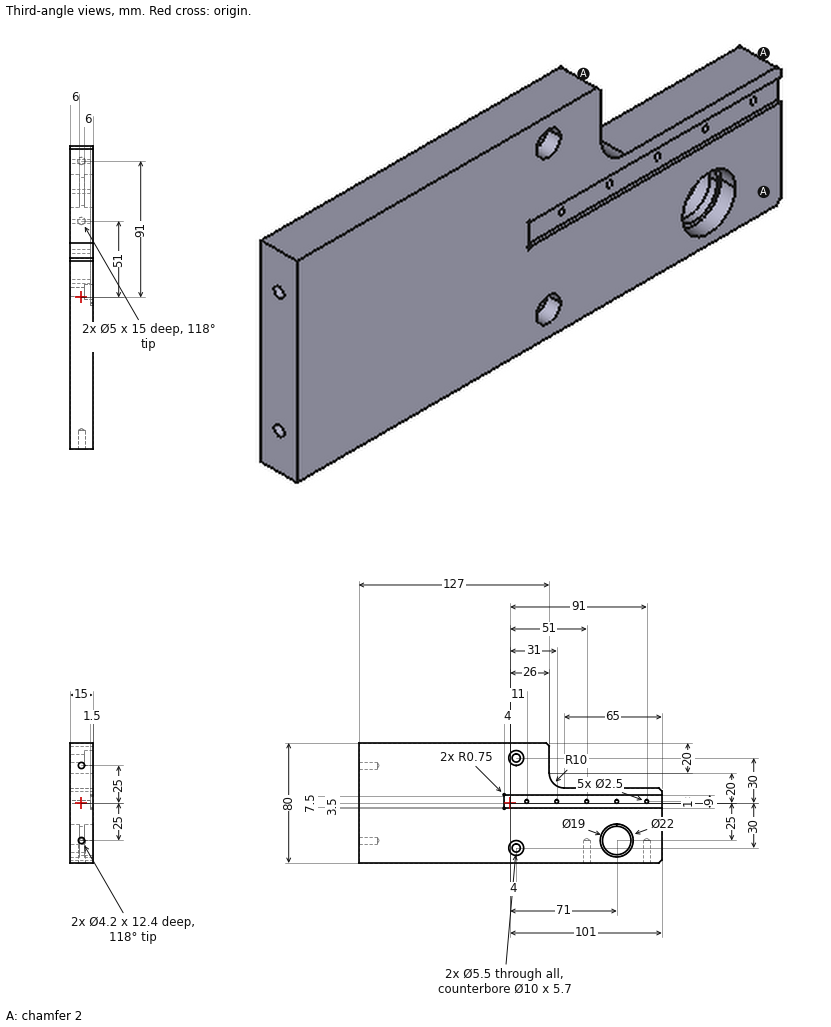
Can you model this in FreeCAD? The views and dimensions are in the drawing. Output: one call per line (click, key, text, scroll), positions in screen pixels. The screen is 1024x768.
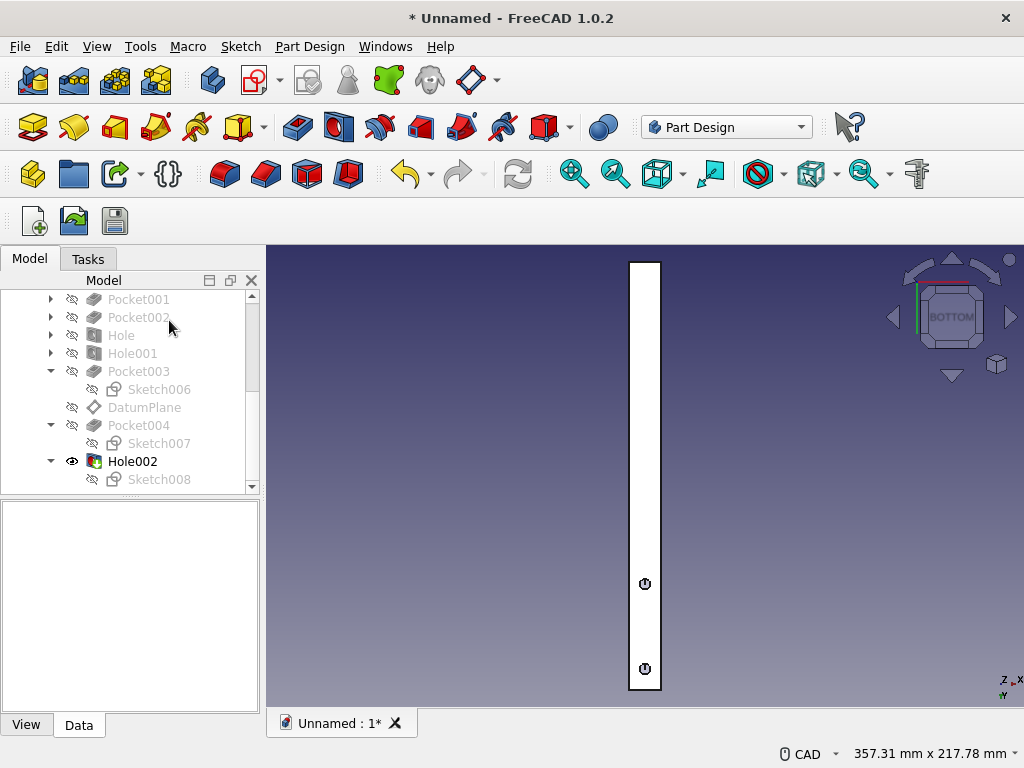
key(0)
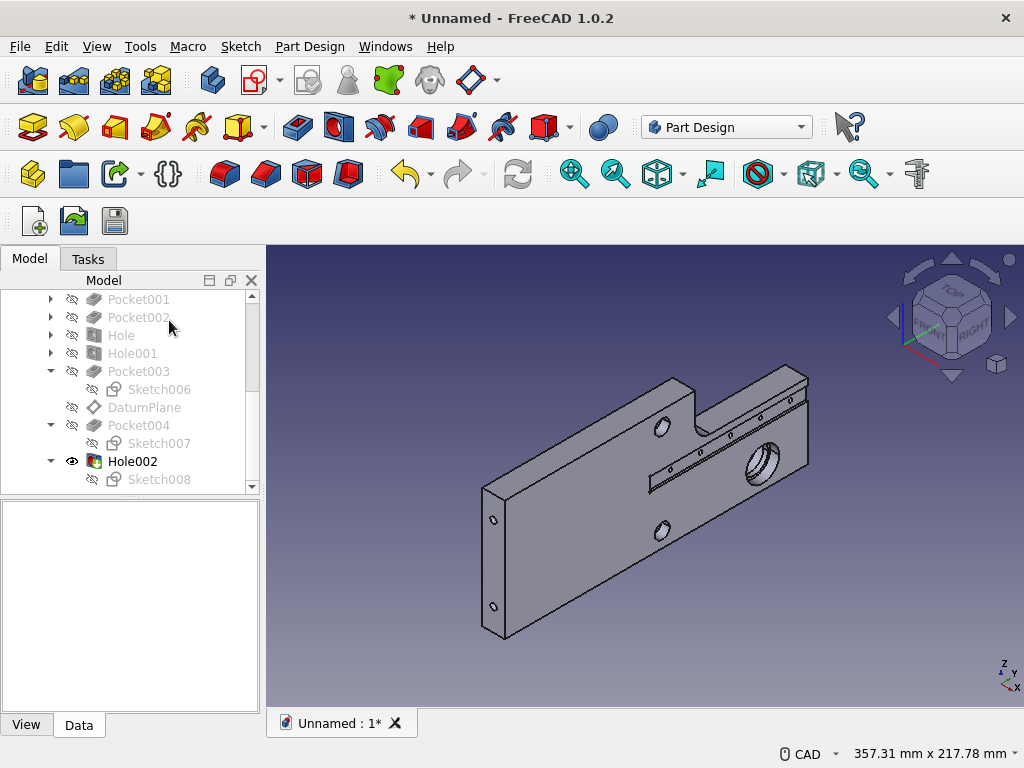
key(2)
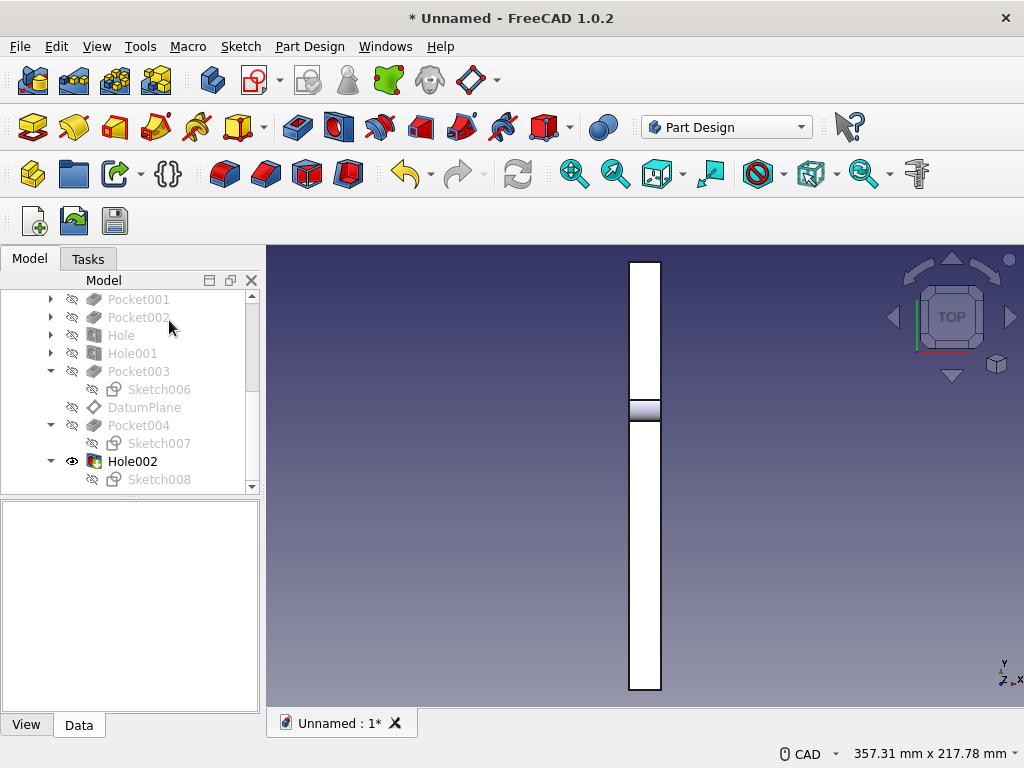
click(645, 420)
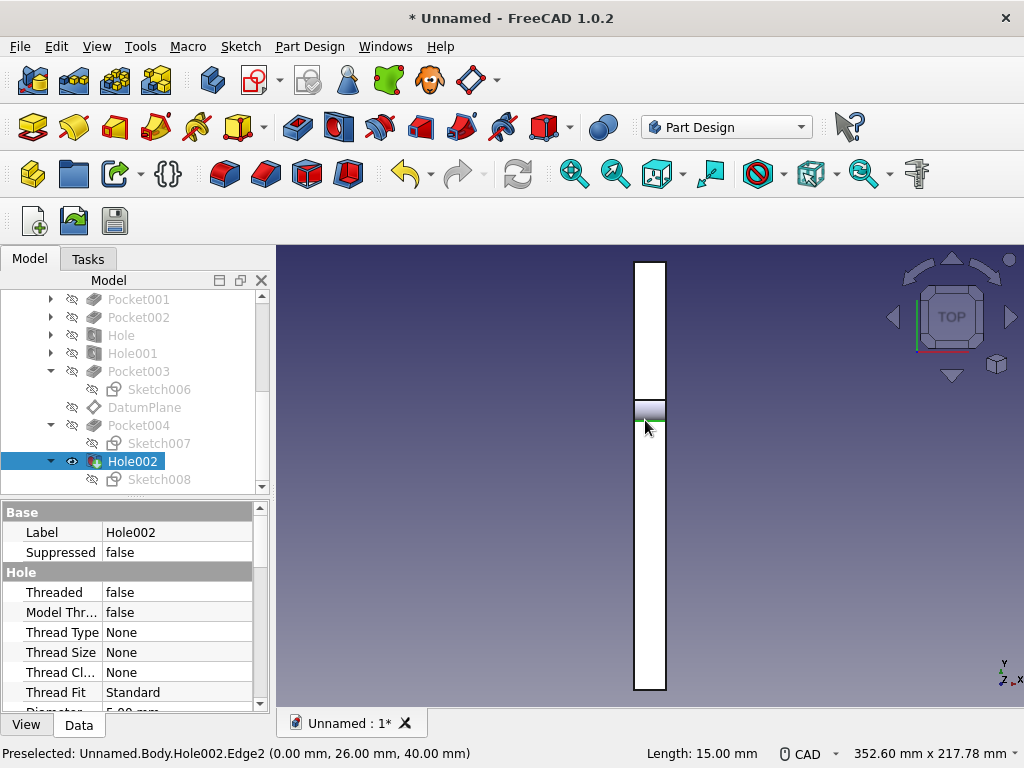
key(1)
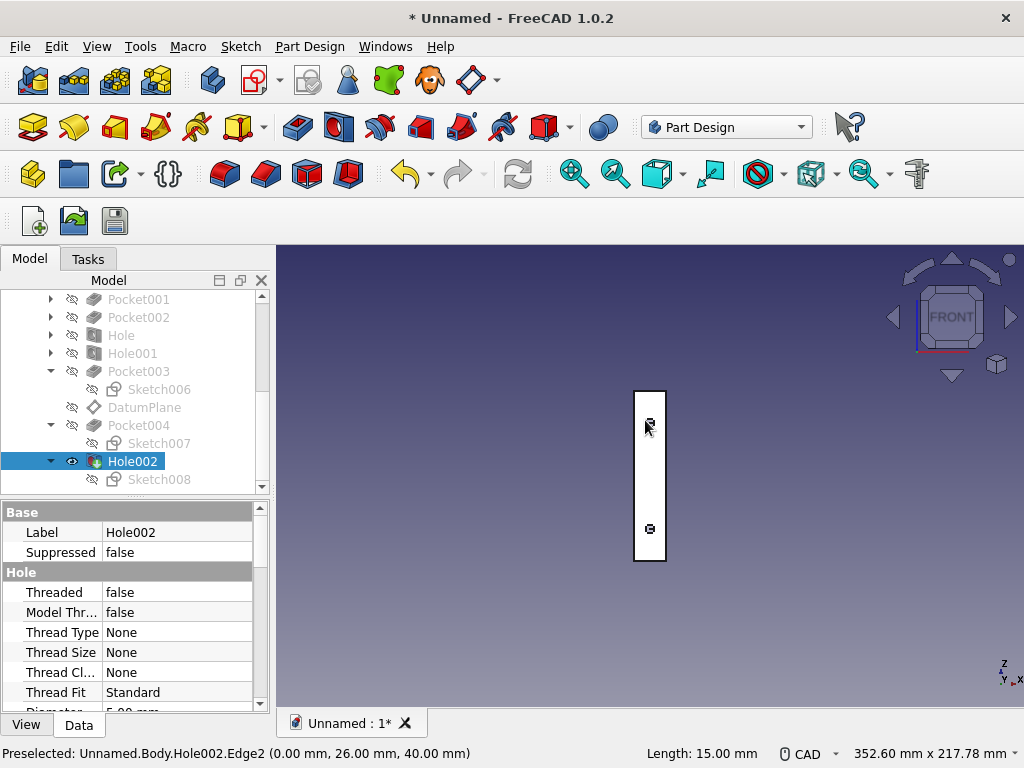
click(575, 174)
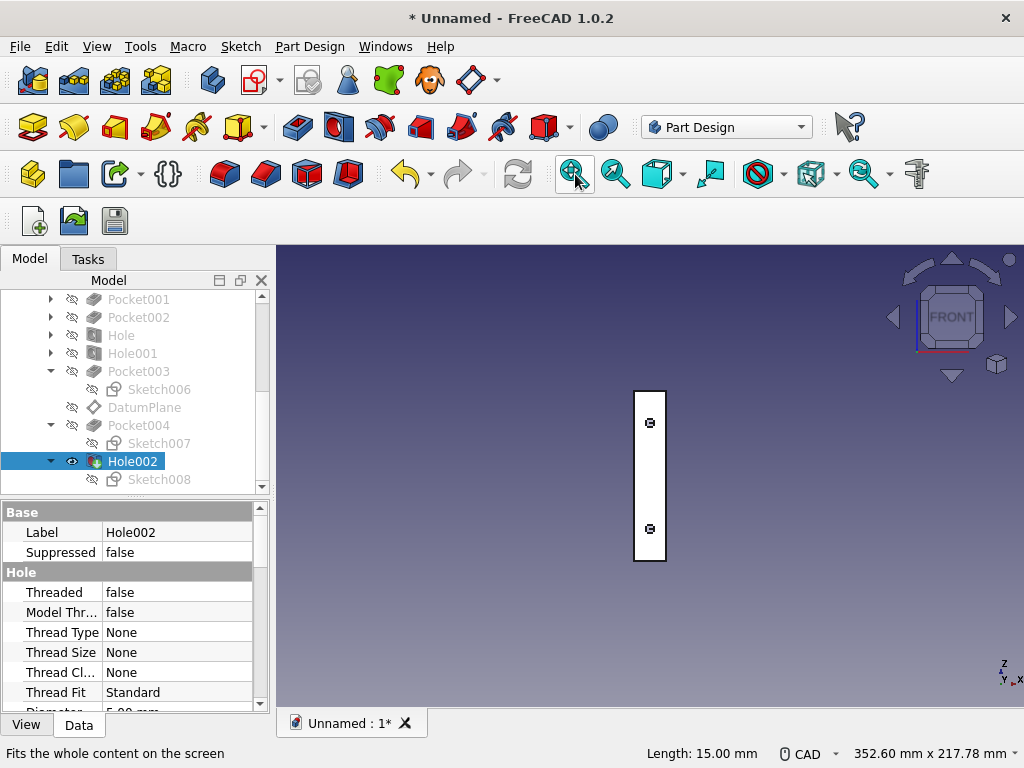
key(3)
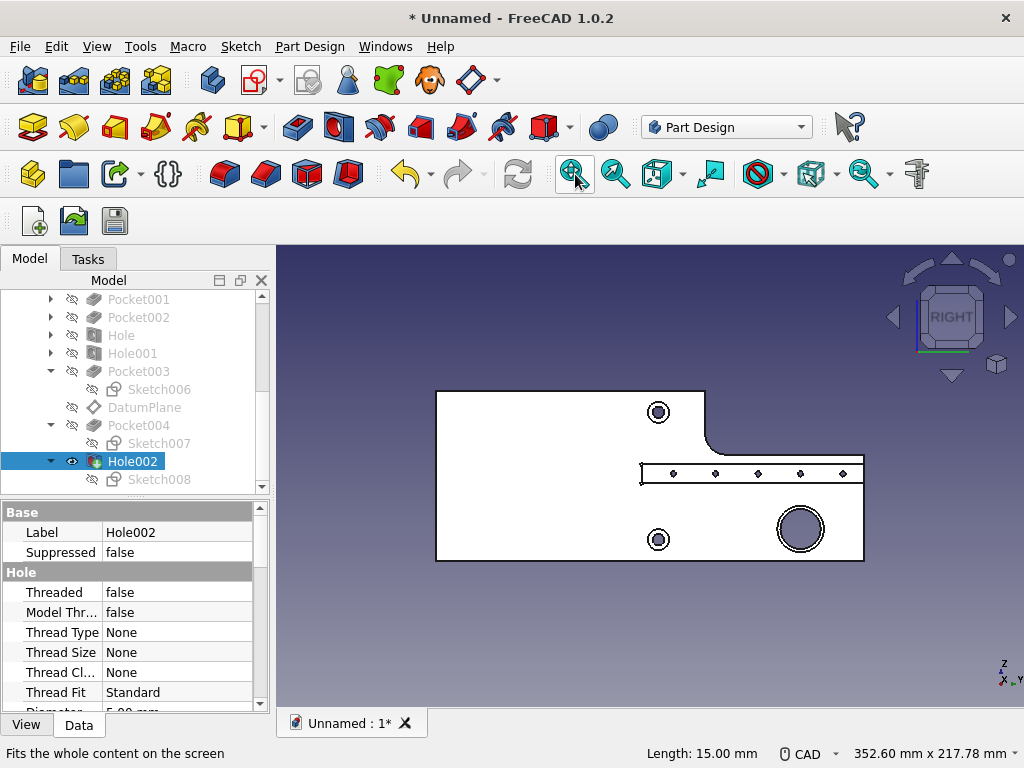
key(5)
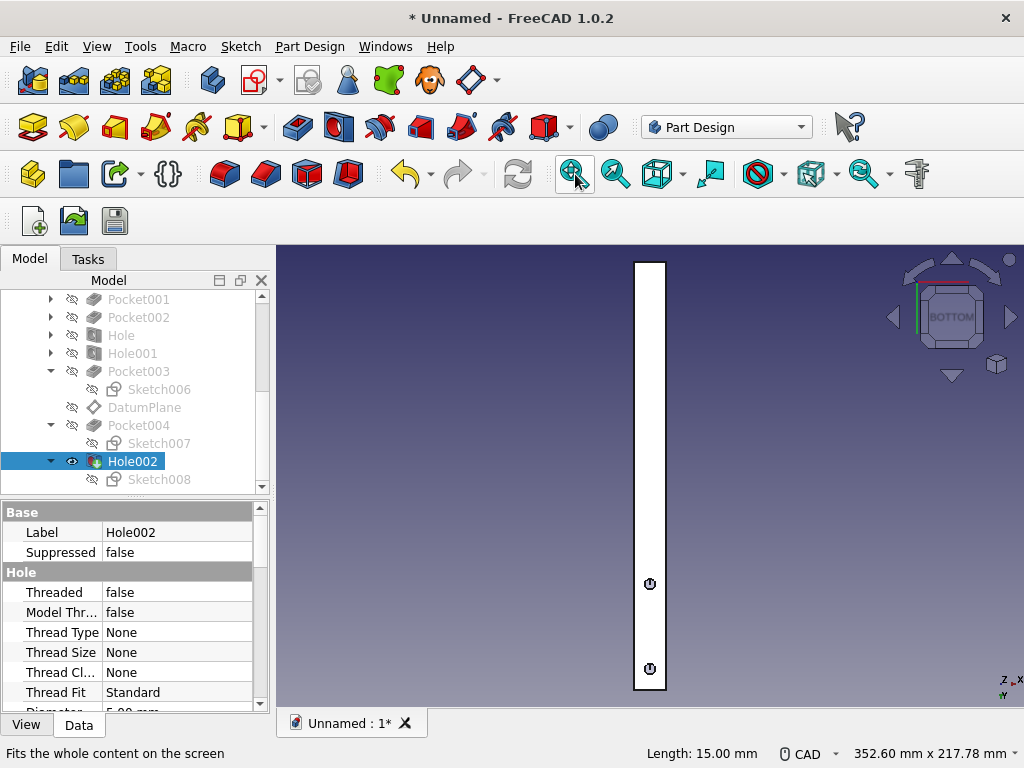
key(4)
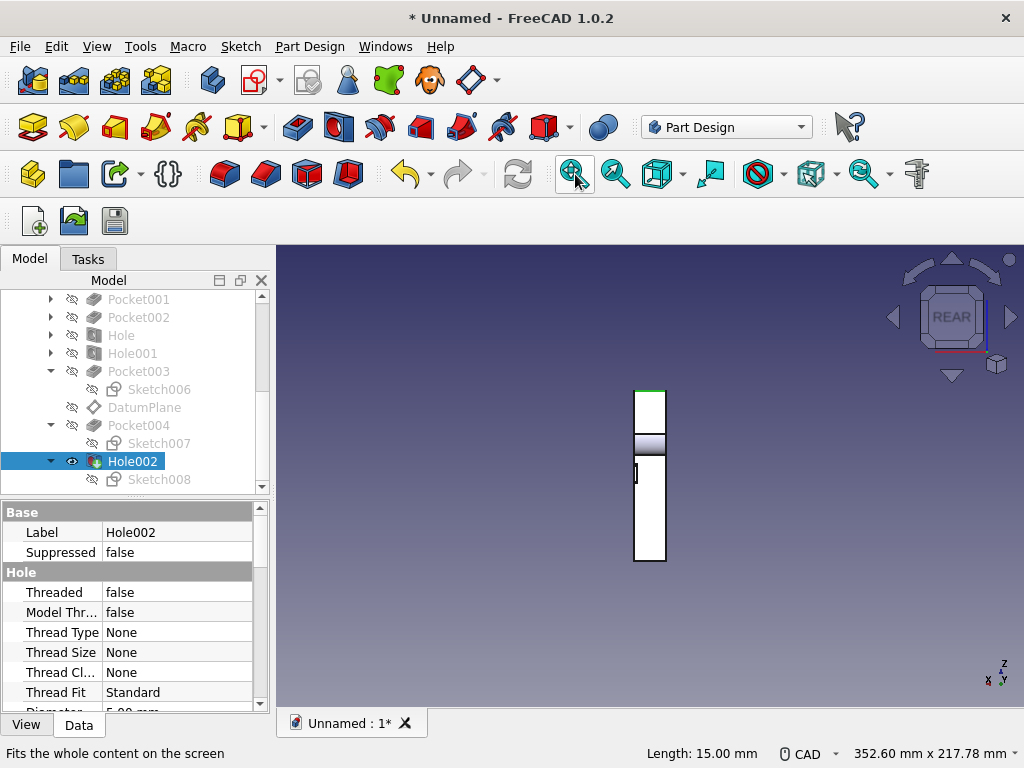
click(575, 174)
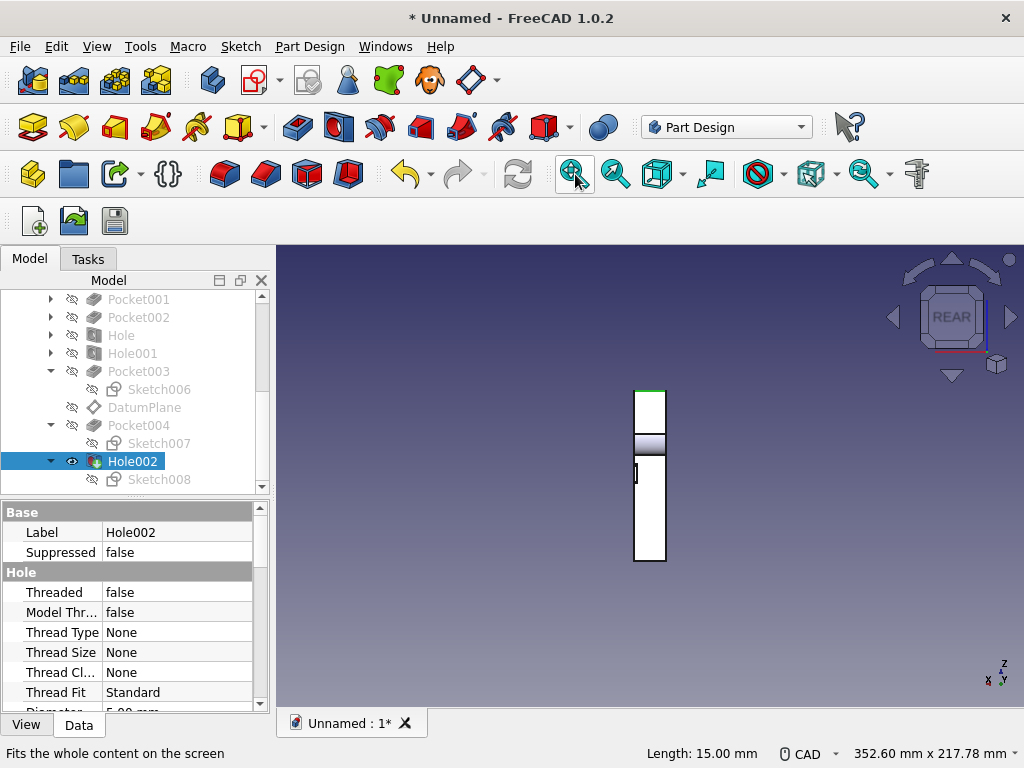
click(650, 454, ctrl)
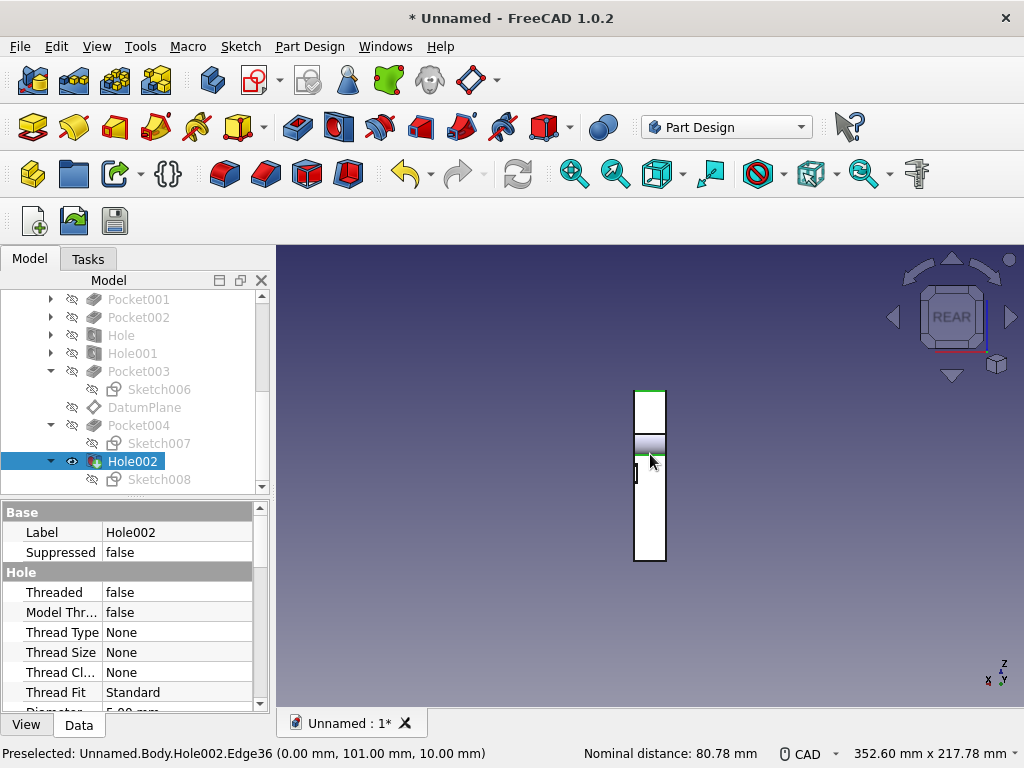
click(650, 560, ctrl)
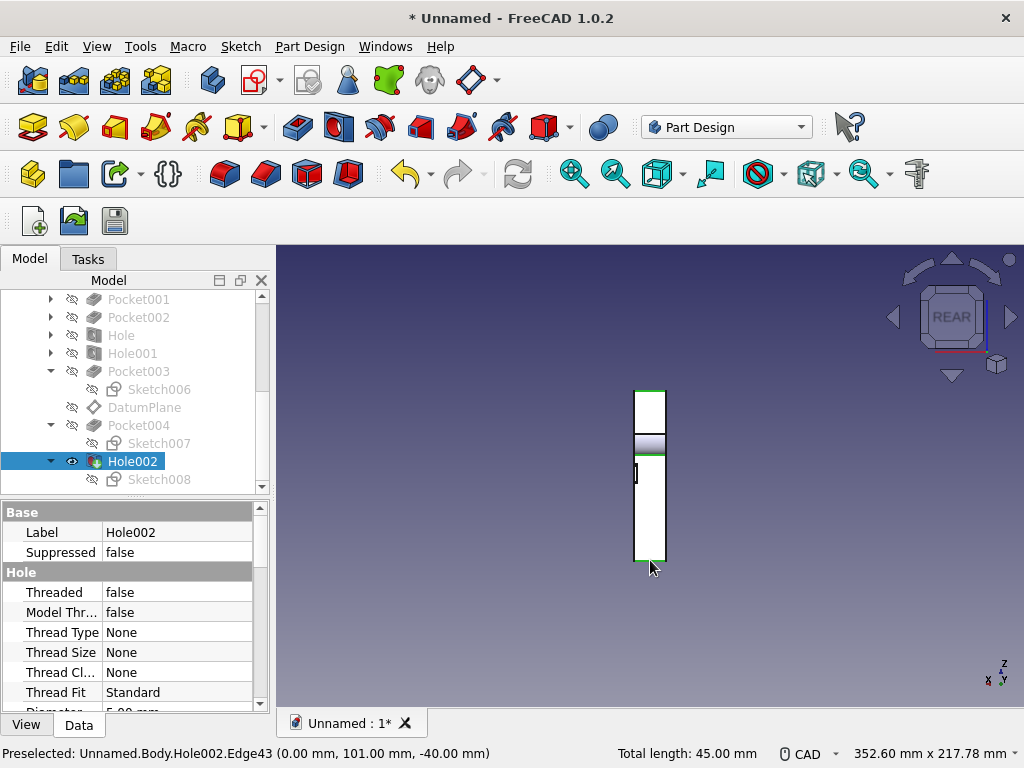
click(266, 174)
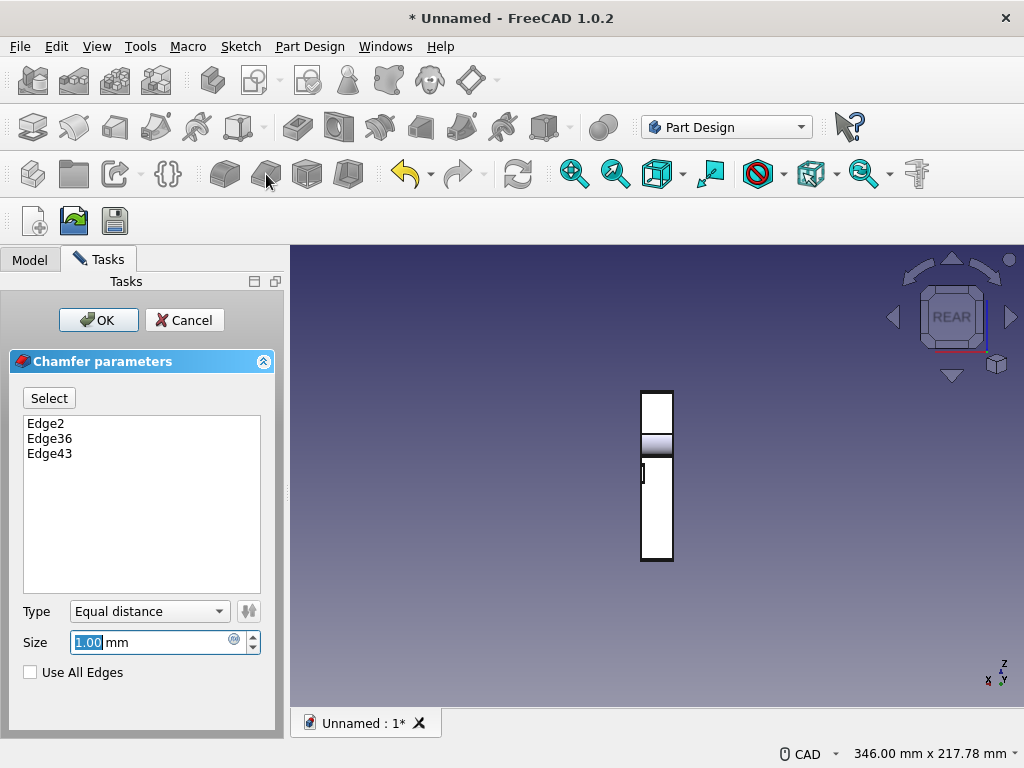
text(2)
key(Tab)